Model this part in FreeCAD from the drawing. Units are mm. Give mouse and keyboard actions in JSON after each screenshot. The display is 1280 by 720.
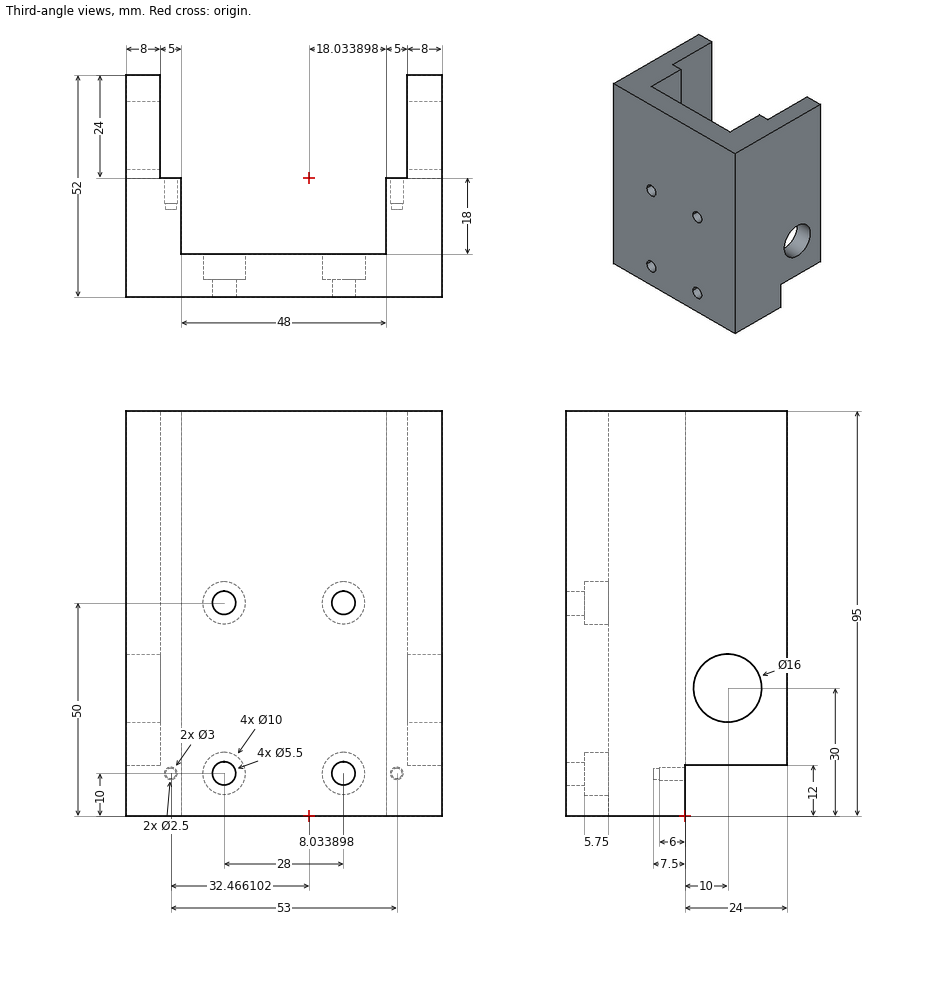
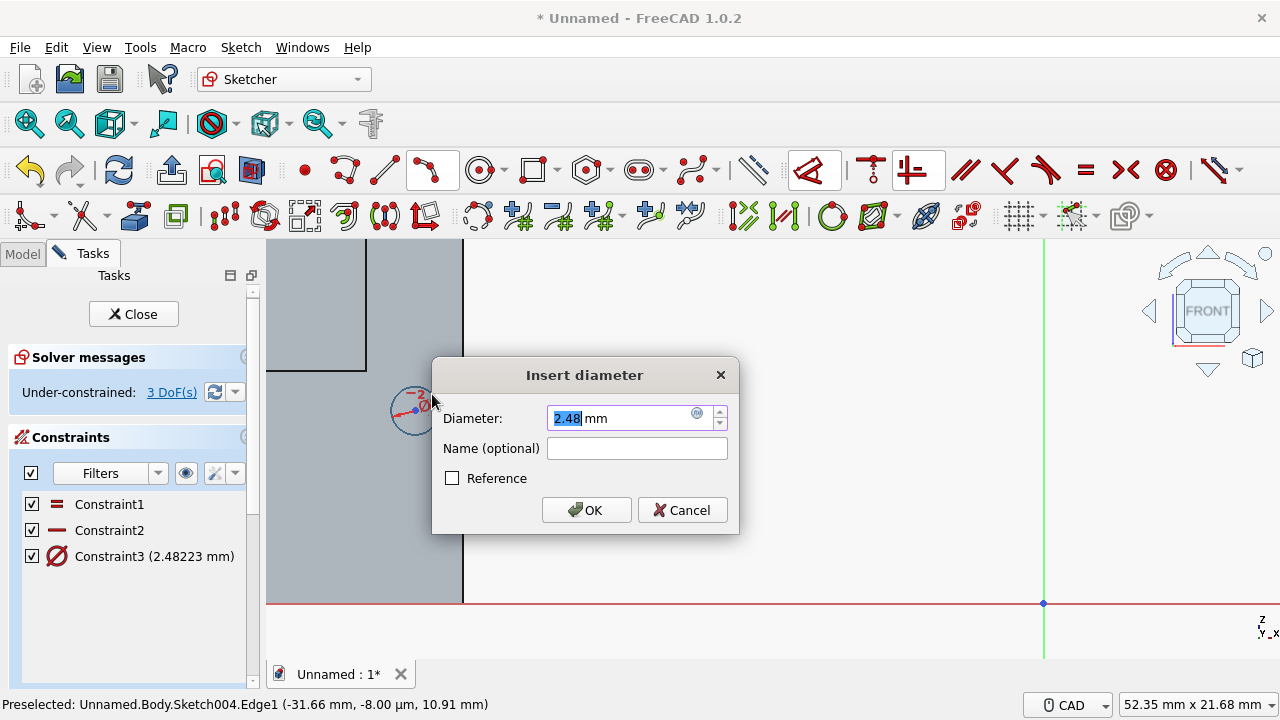
{"action": "type", "text": "2.5"}
{"action": "key", "text": "Return"}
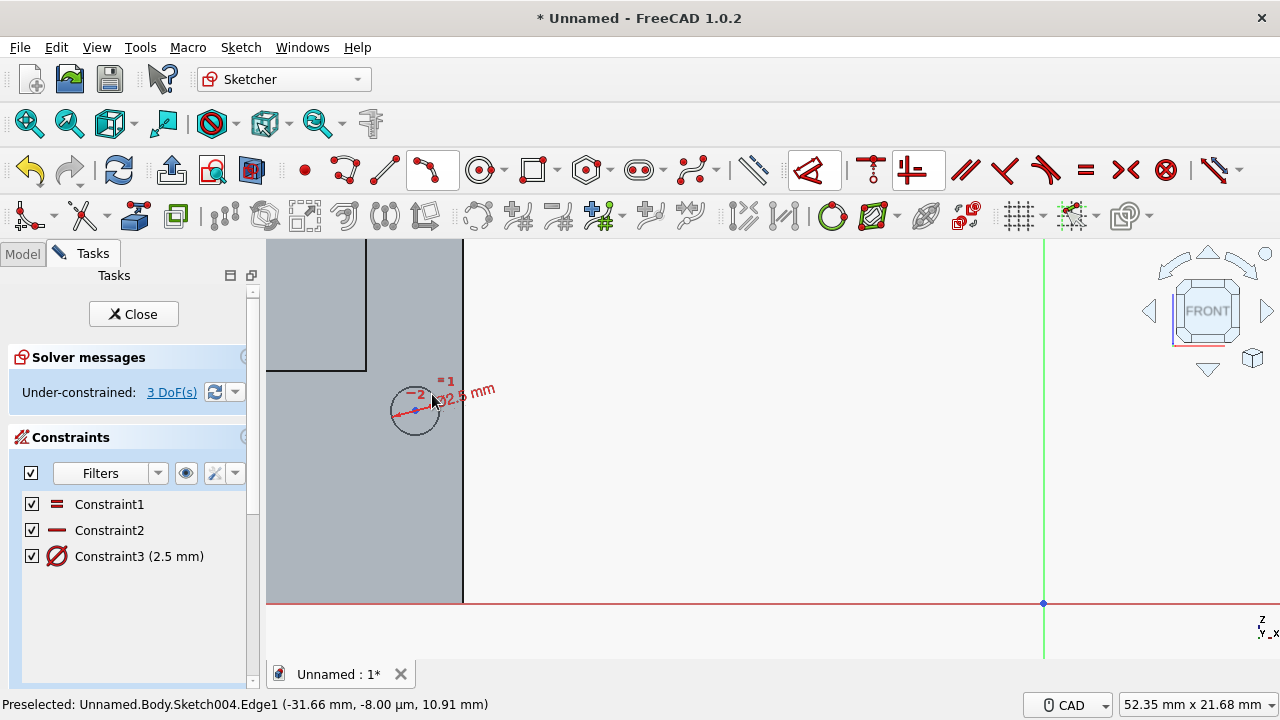
{"action": "left_click", "coordinate": [415, 411]}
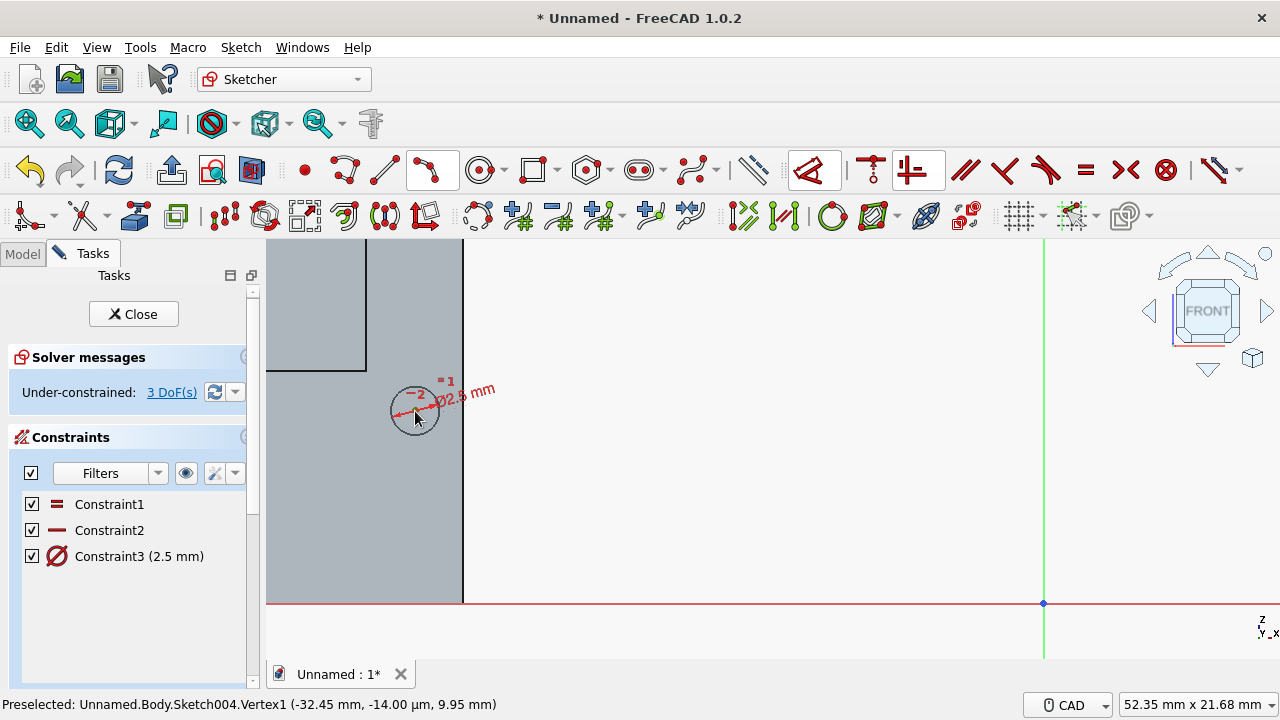
{"action": "key", "text": "i"}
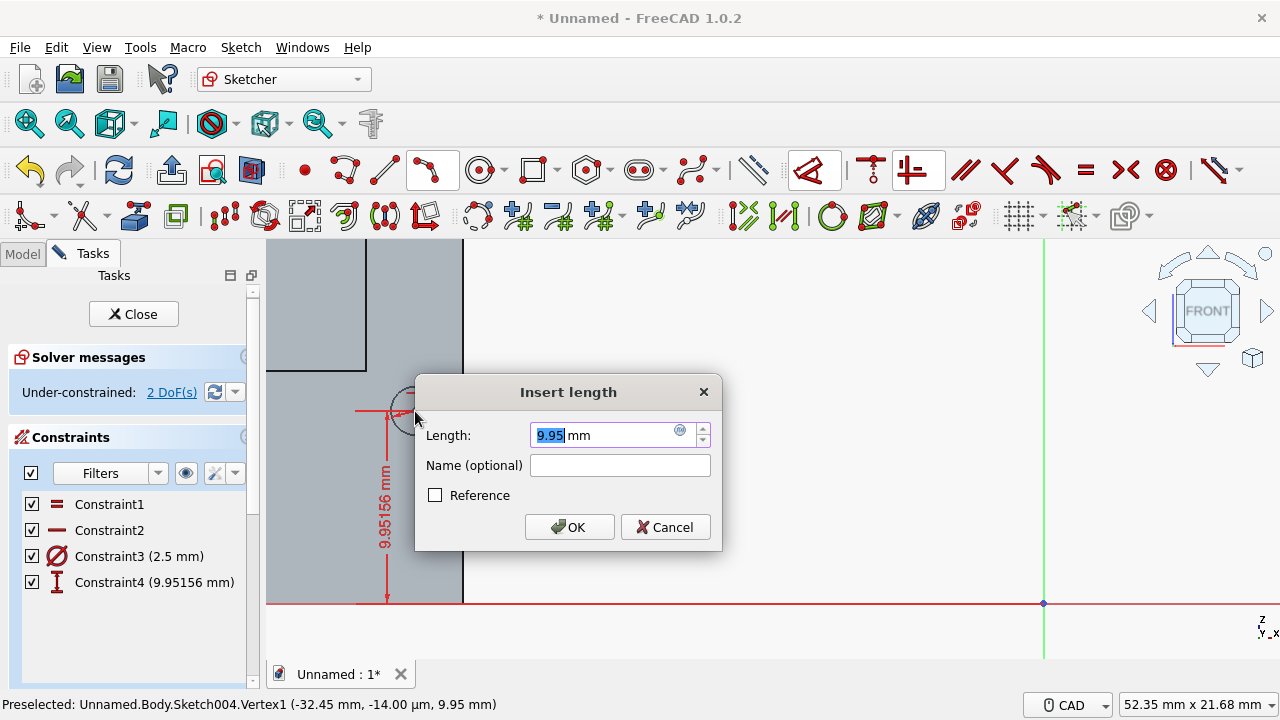
{"action": "type", "text": "10"}
{"action": "key", "text": "Return"}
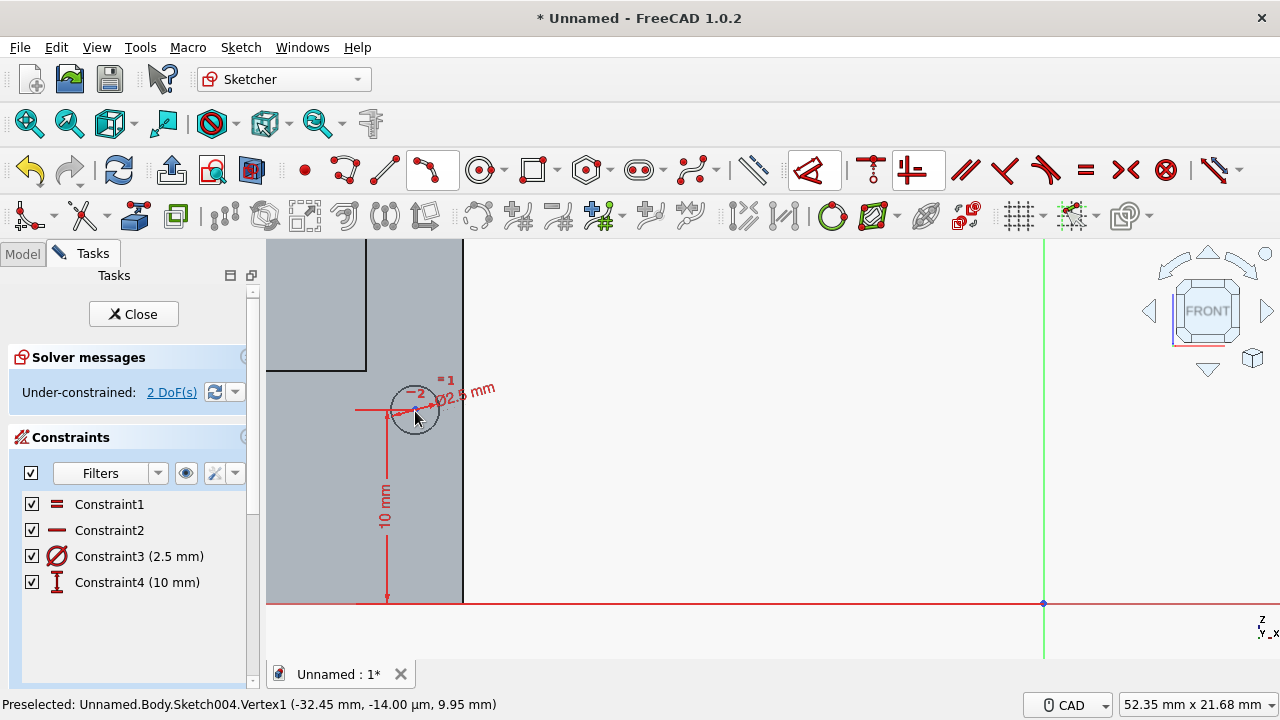
{"action": "left_click", "coordinate": [415, 410]}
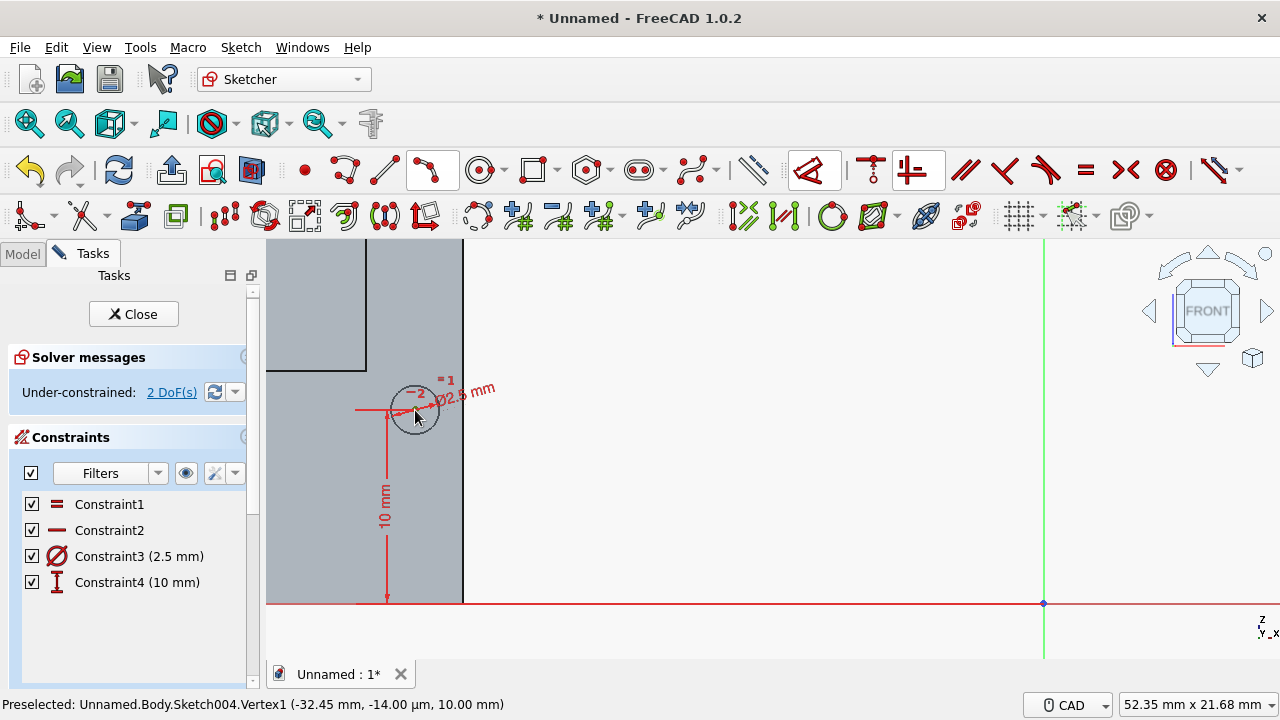
{"action": "scroll", "coordinate": [432, 394], "scroll_direction": "down", "scroll_amount": 3}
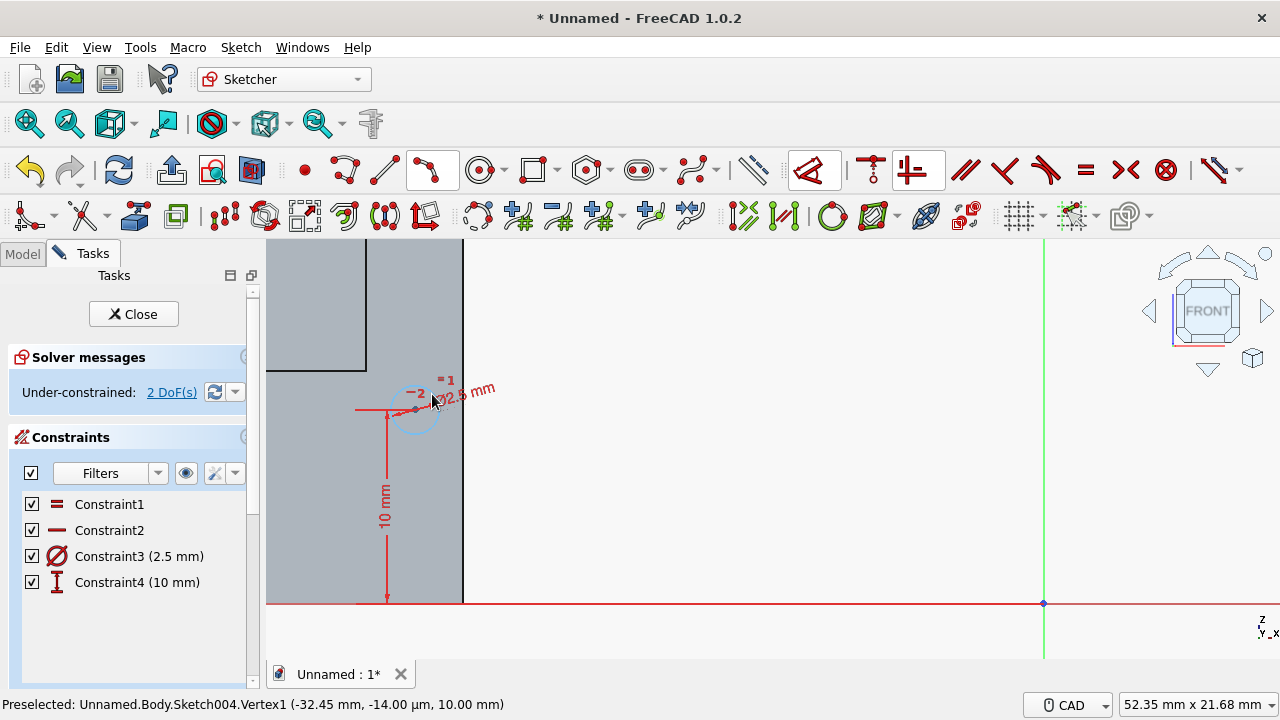
{"action": "left_click", "coordinate": [986, 403]}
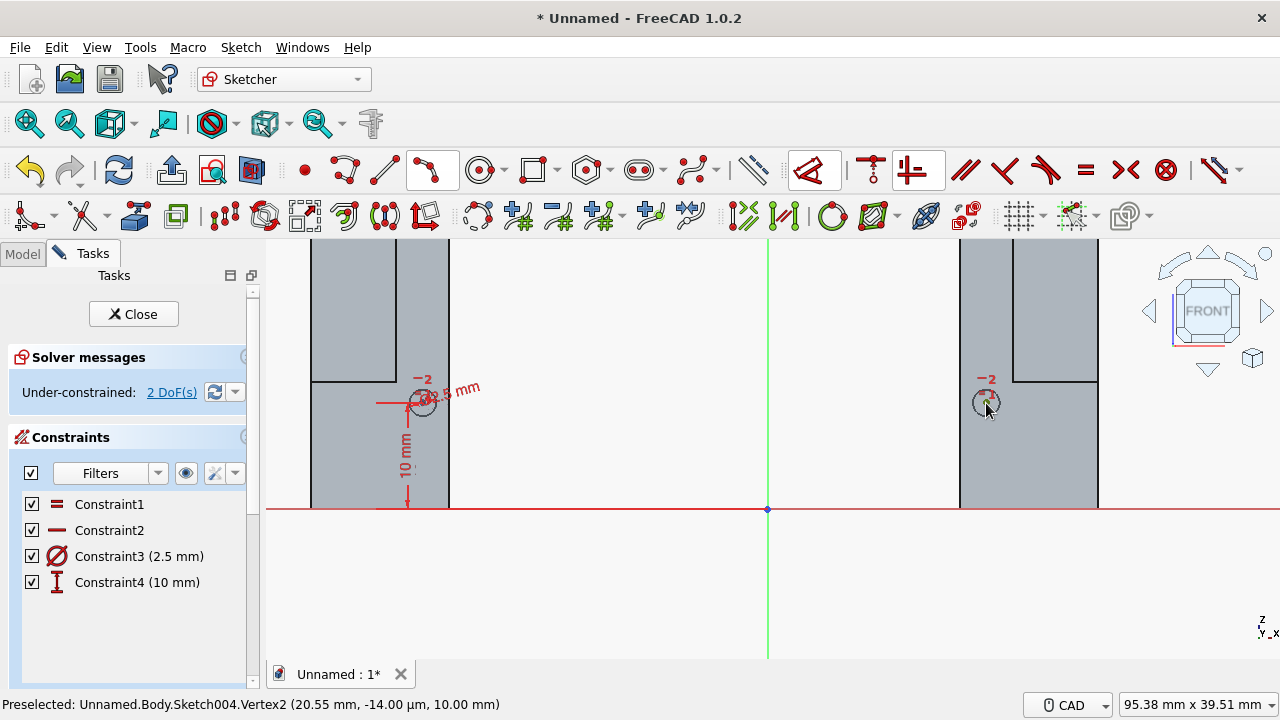
{"action": "key", "text": "l"}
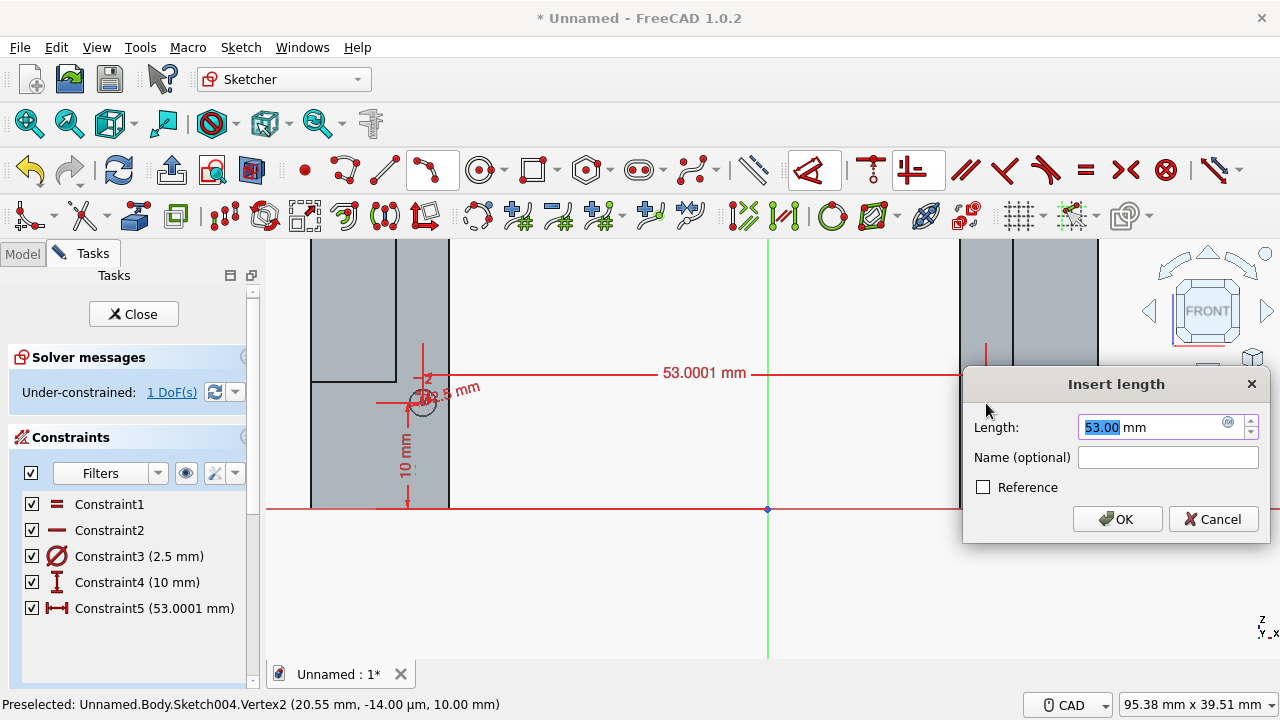
{"action": "type", "text": "53"}
{"action": "key", "text": "Return"}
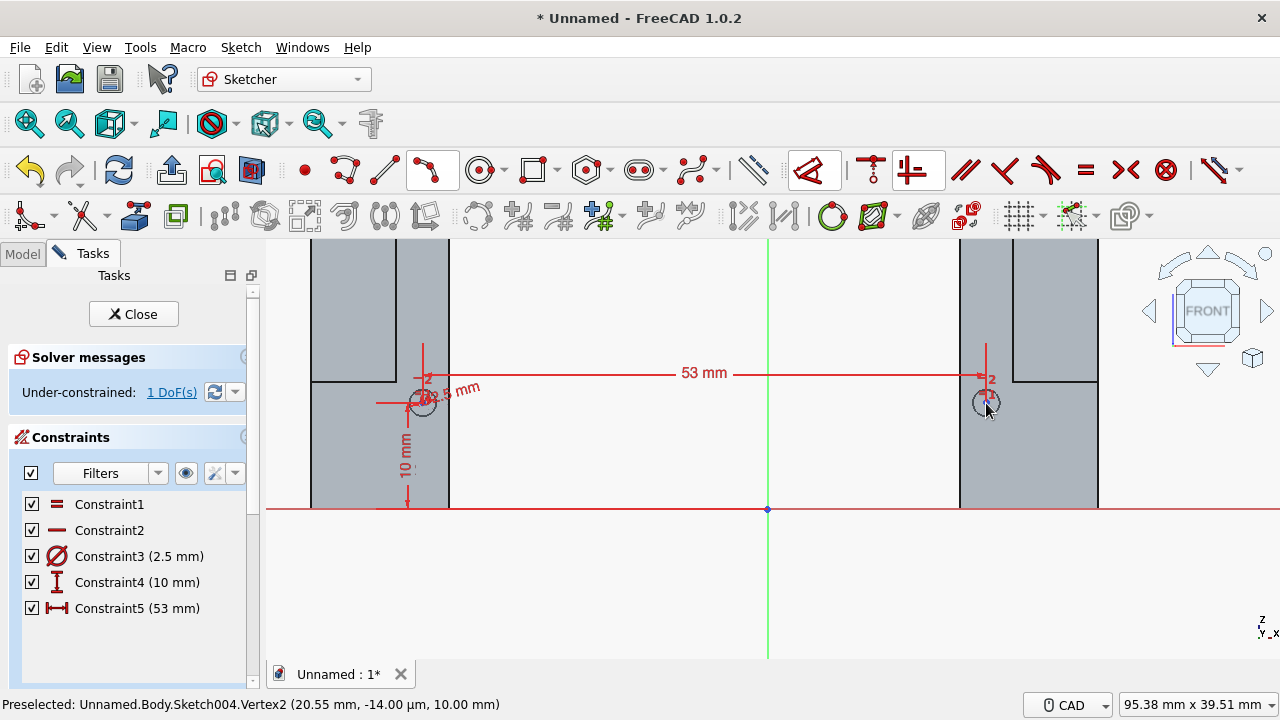
{"action": "left_click", "coordinate": [423, 403]}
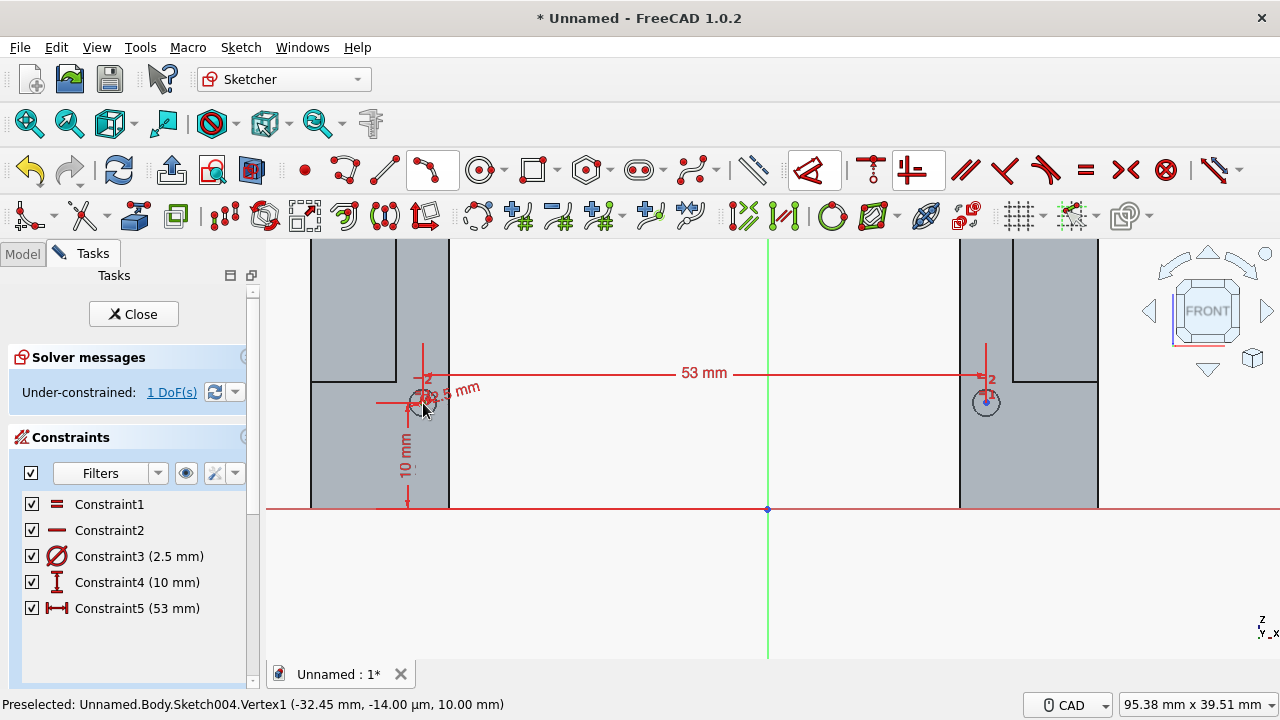
{"action": "left_click", "coordinate": [836, 170]}